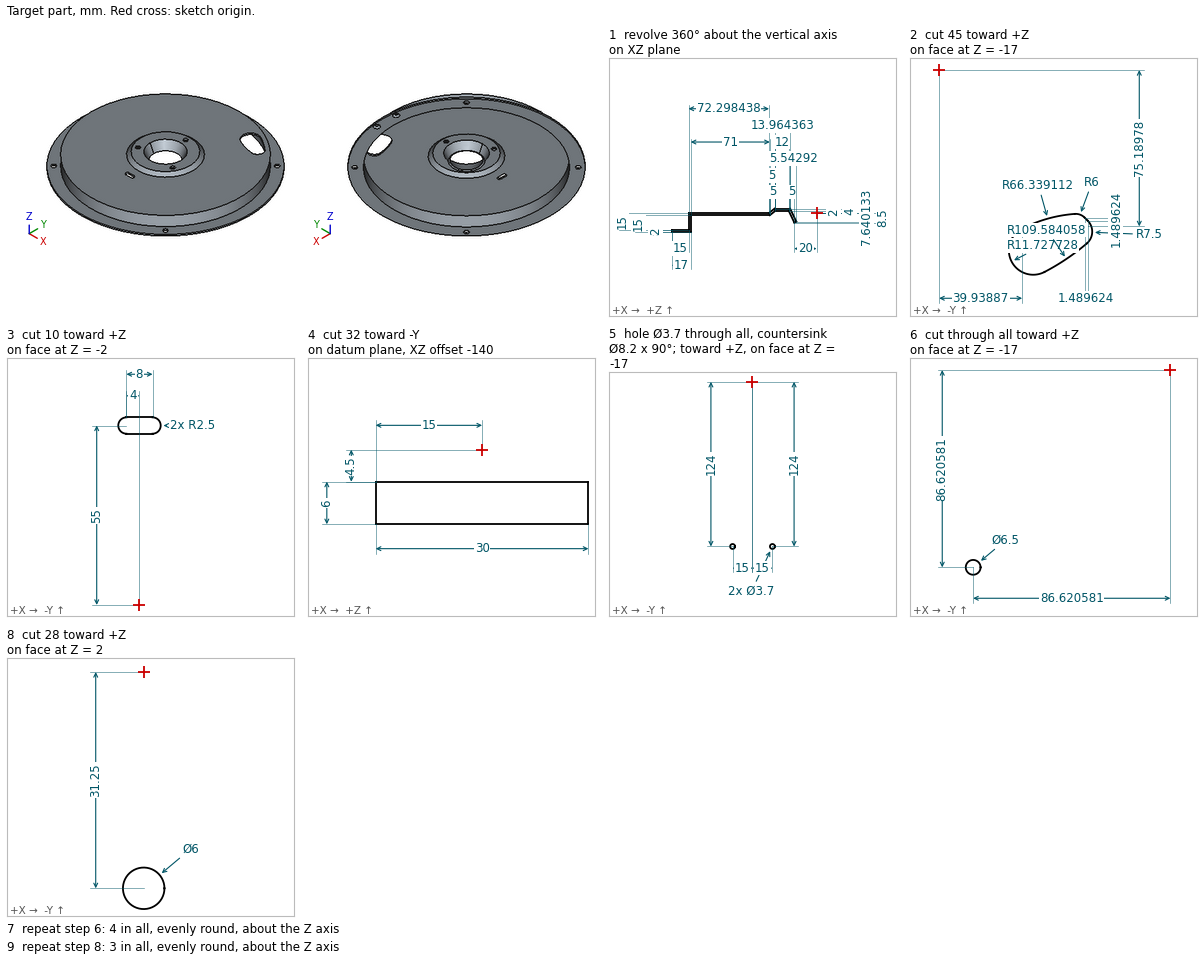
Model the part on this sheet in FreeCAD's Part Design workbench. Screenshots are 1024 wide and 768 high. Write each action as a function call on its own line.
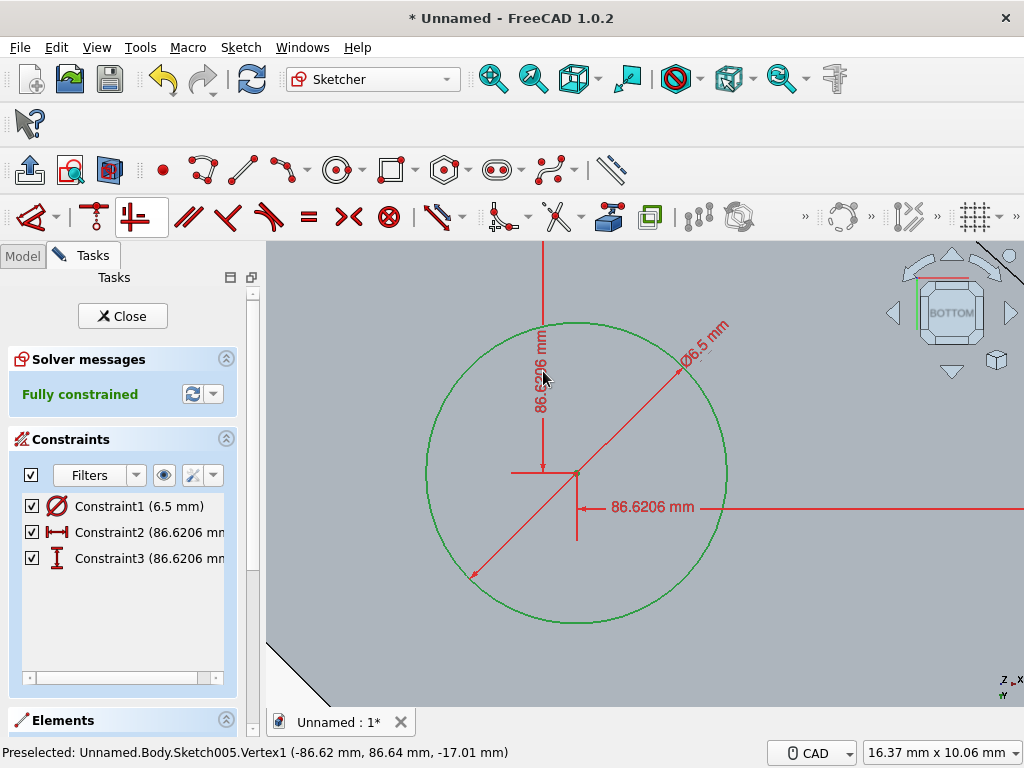
click(123, 316)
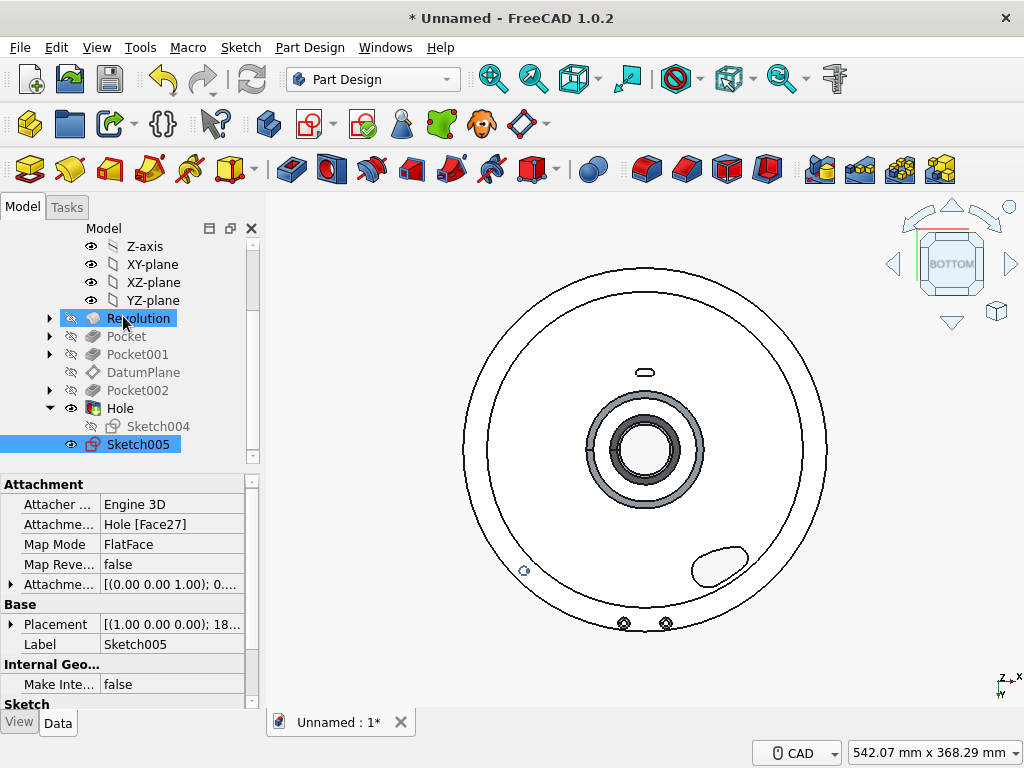
click(292, 170)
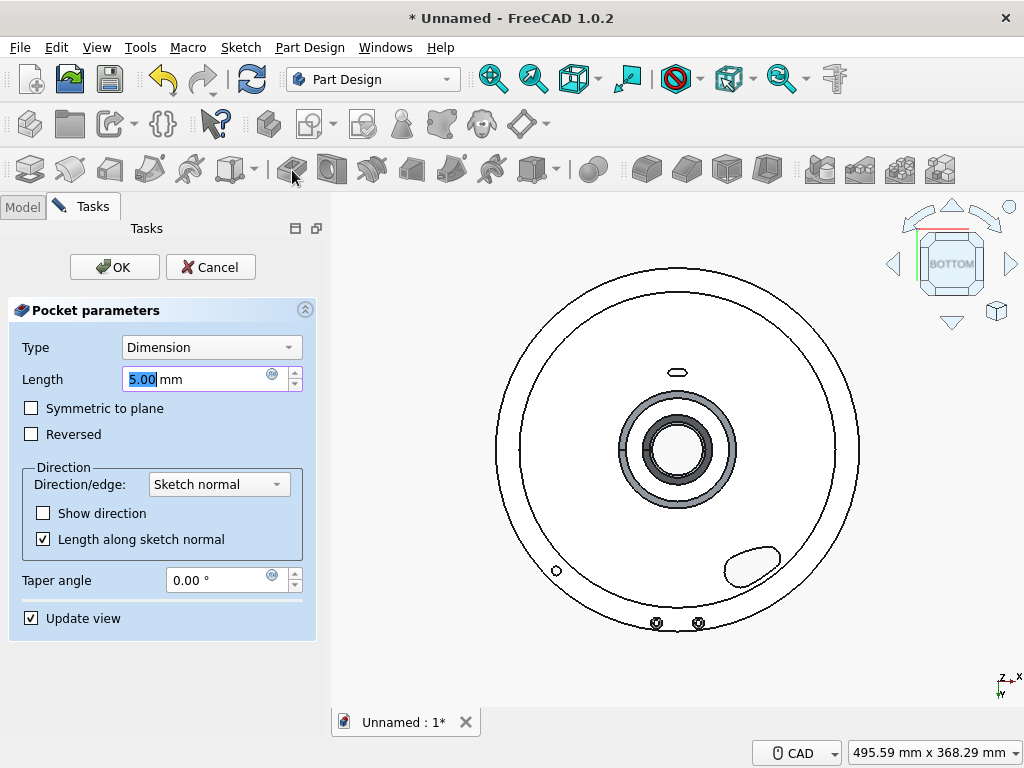
click(212, 348)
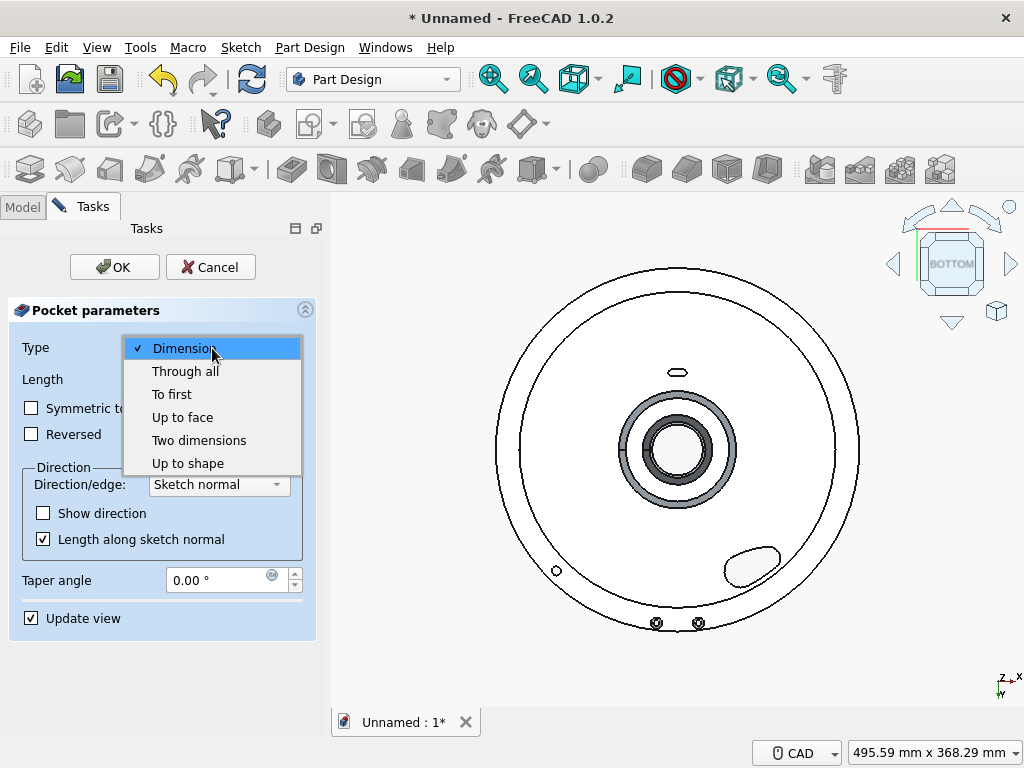
click(212, 372)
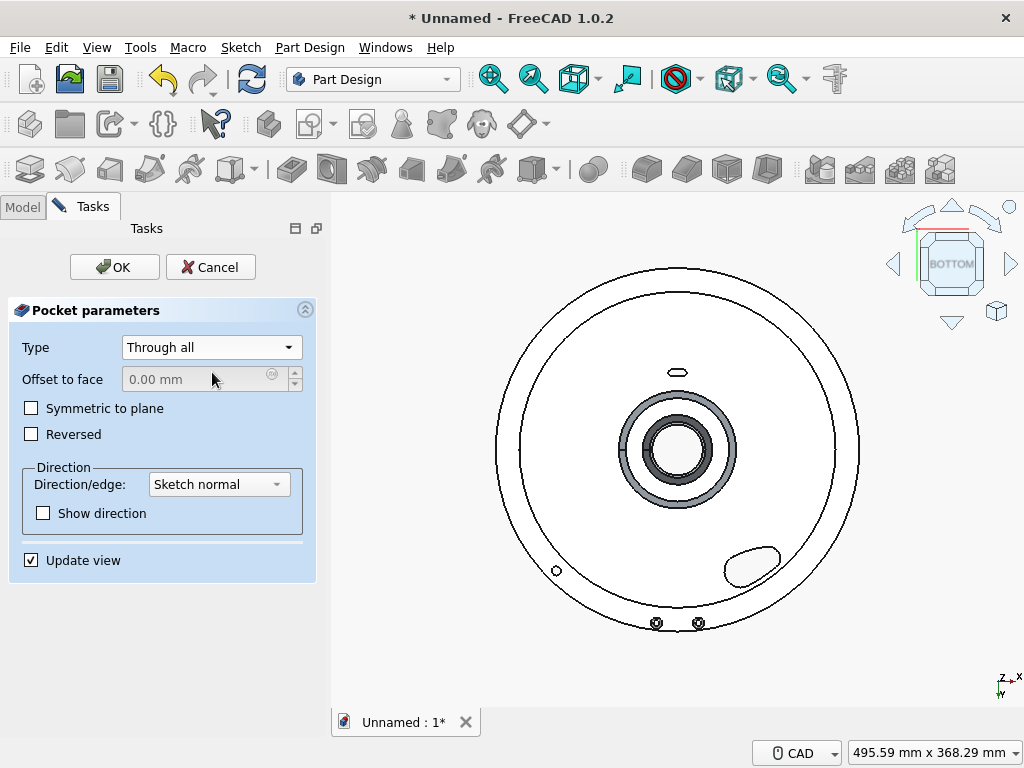
click(115, 267)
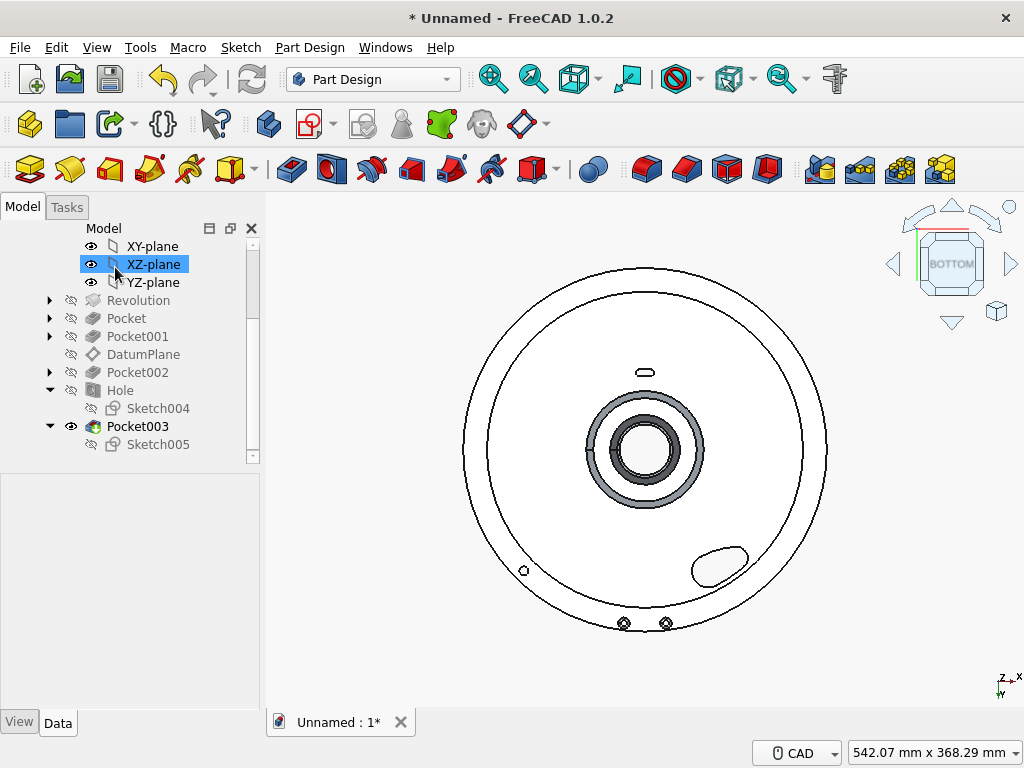
click(116, 426)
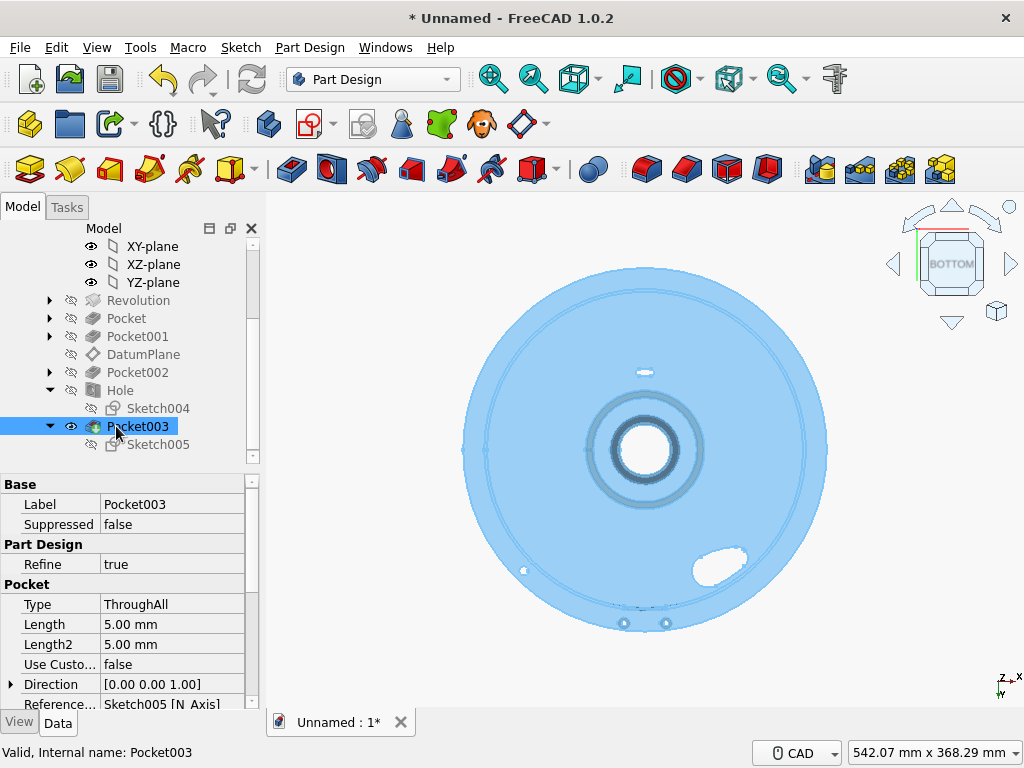
click(900, 170)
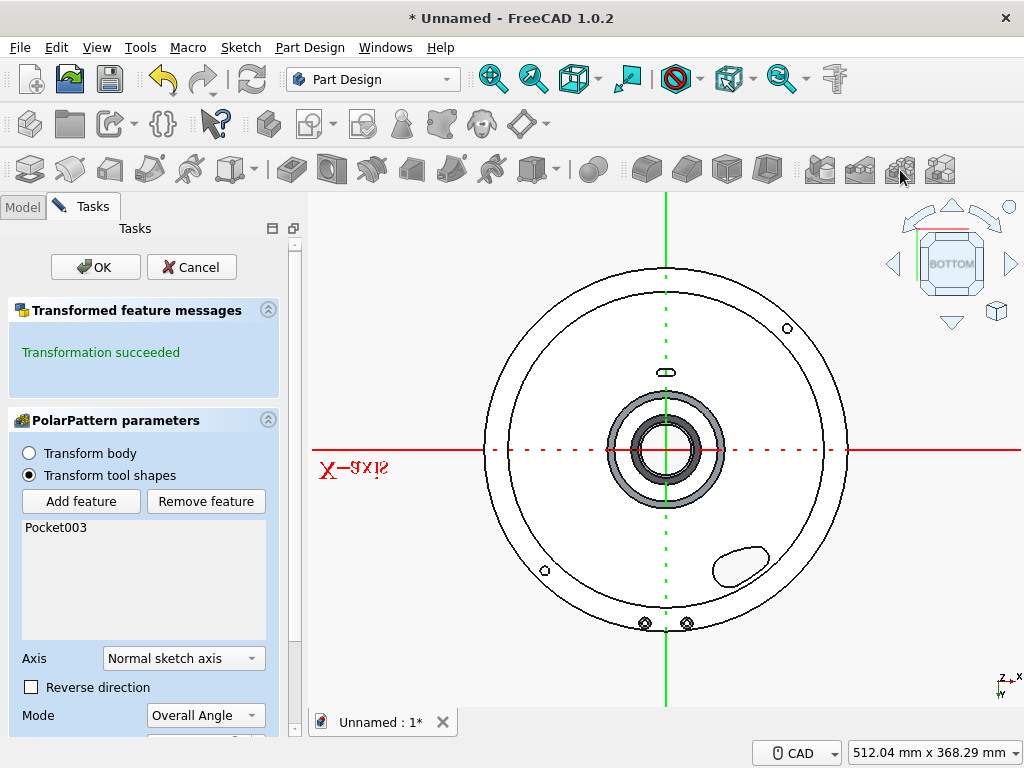
click(184, 658)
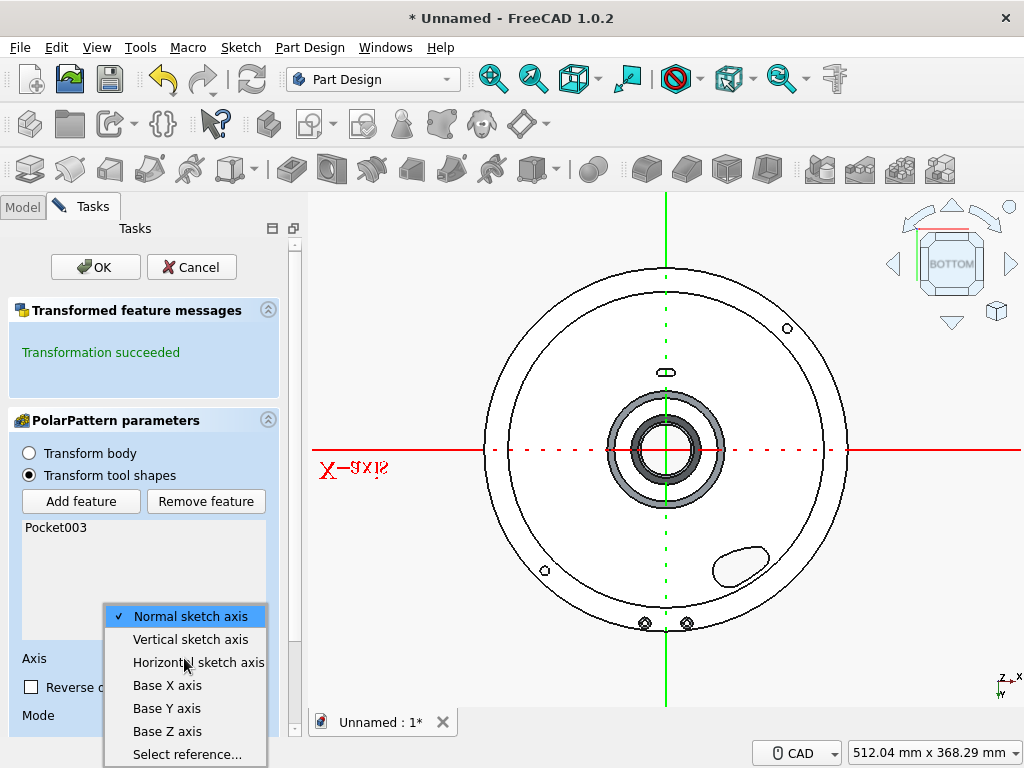
click(184, 732)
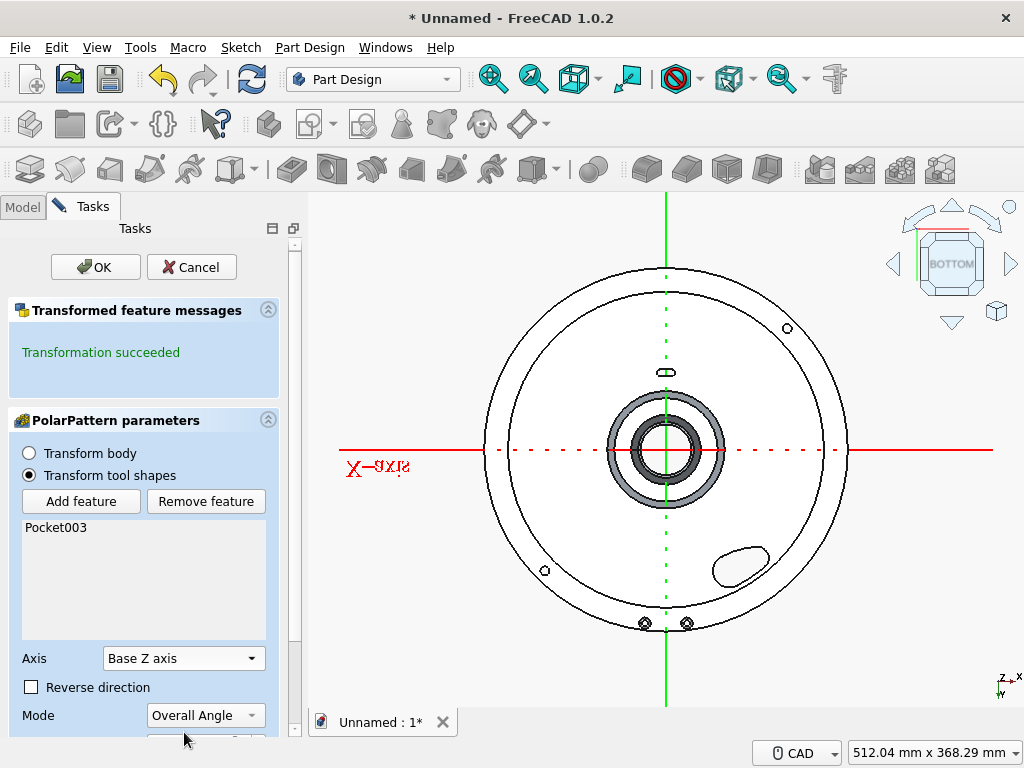
scroll(295, 487, down, 2)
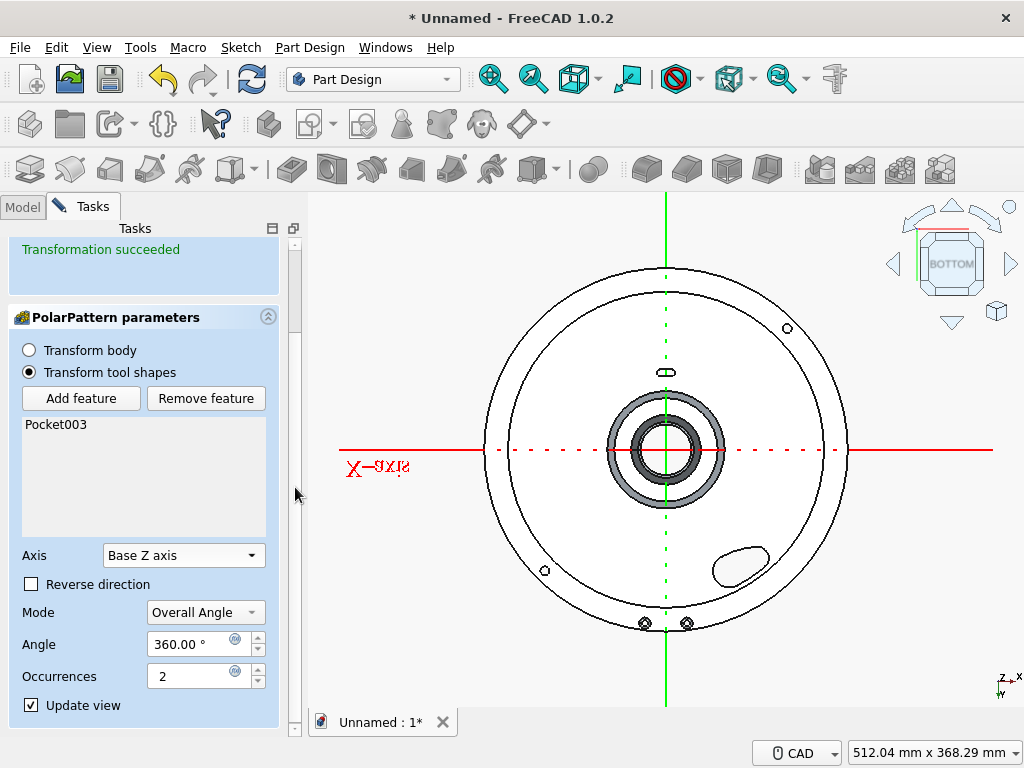
triple_click(198, 676)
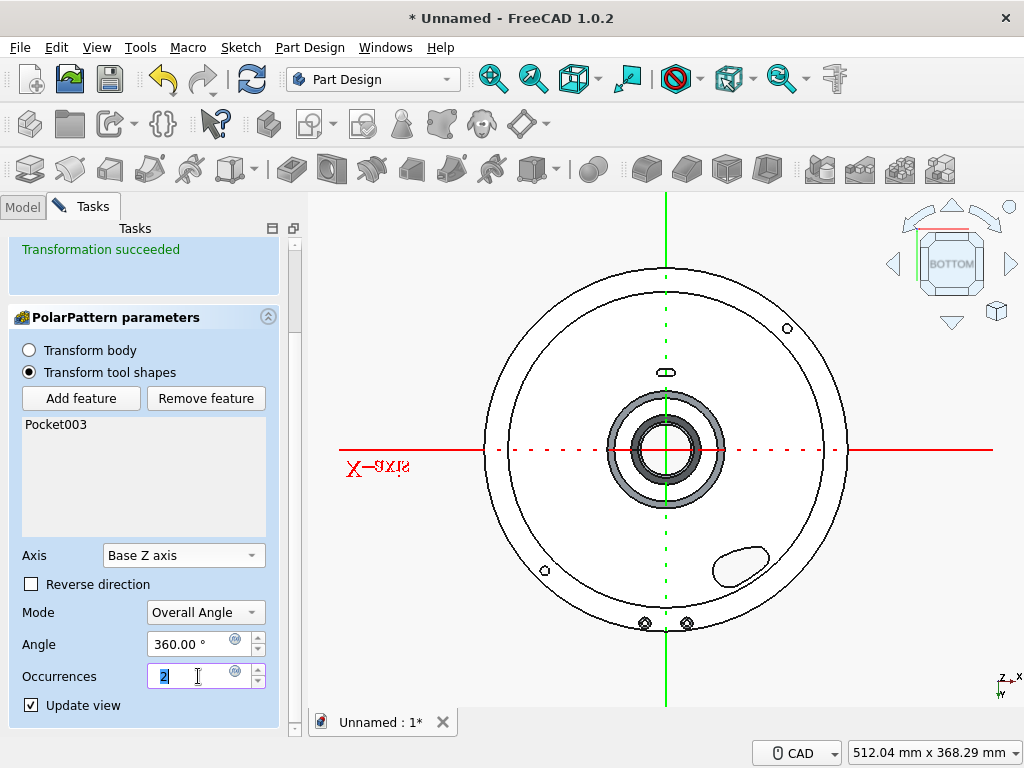
text(4)
key(Tab)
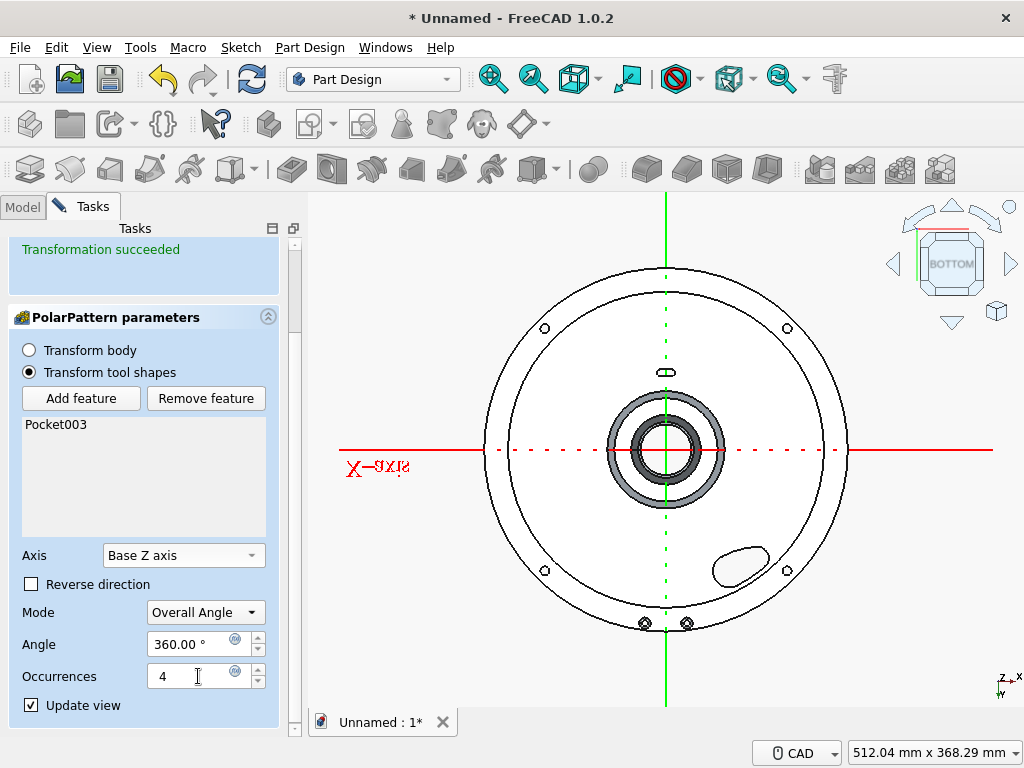
scroll(295, 487, up, 3)